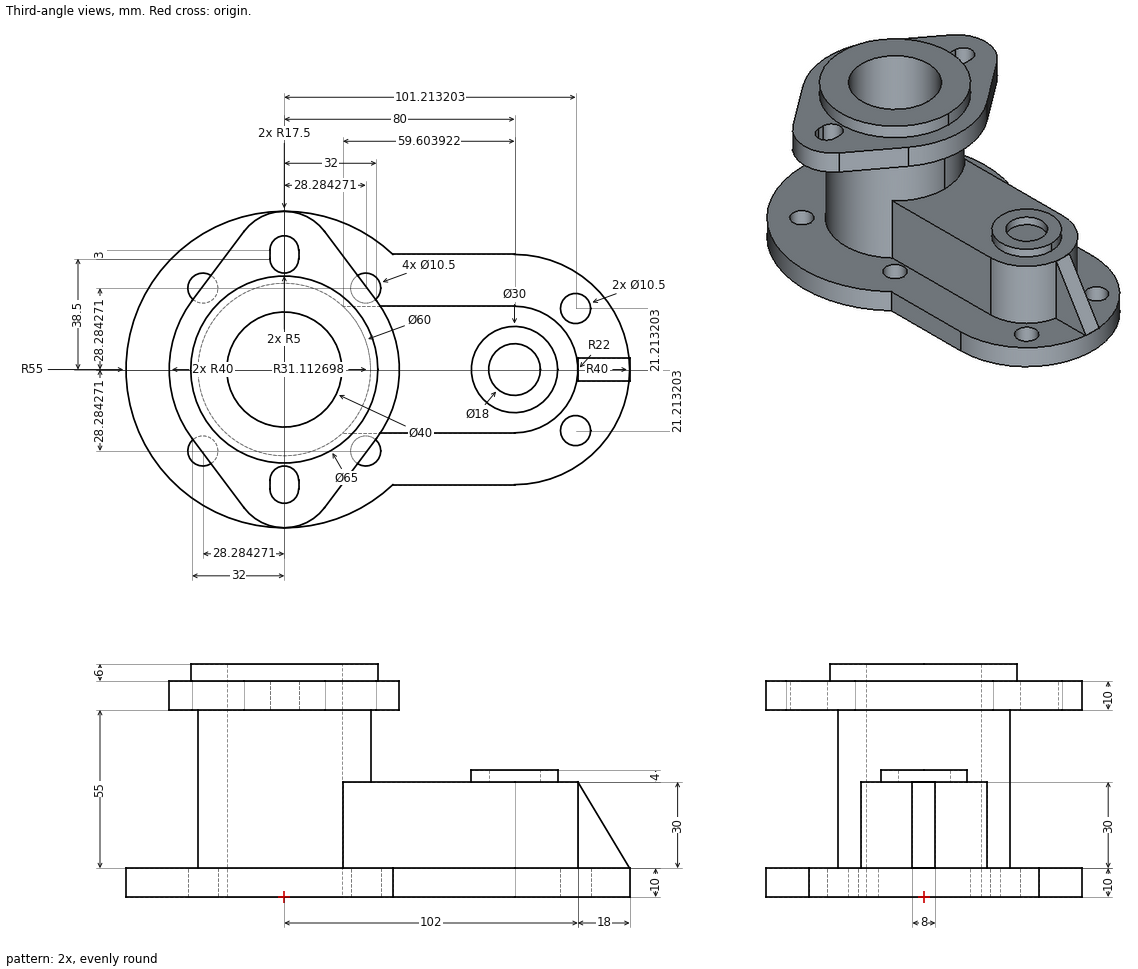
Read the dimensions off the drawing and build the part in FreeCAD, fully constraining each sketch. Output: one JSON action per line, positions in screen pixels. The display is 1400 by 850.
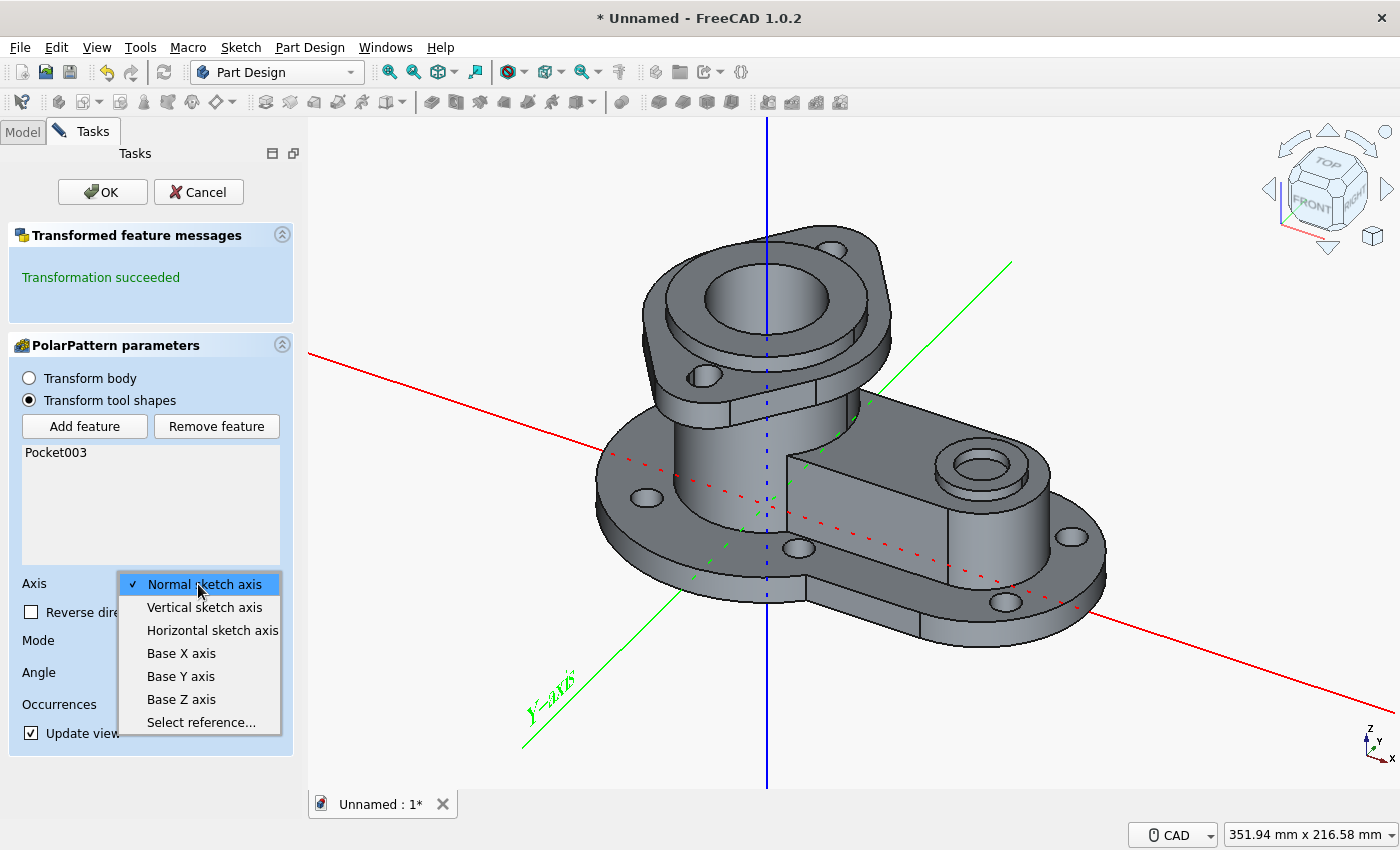
{"action": "left_click", "coordinate": [198, 700]}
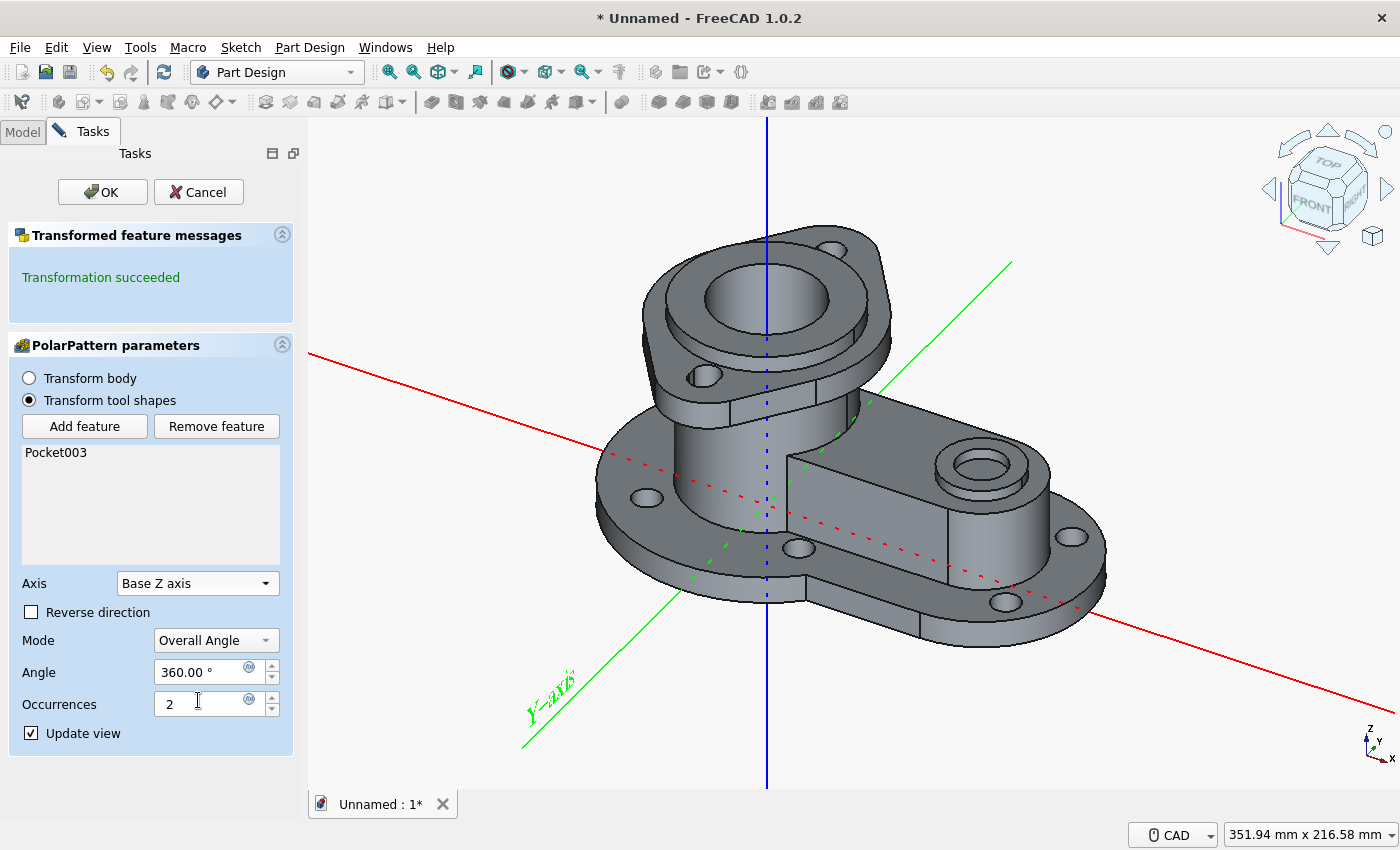
{"action": "triple_click", "coordinate": [209, 704]}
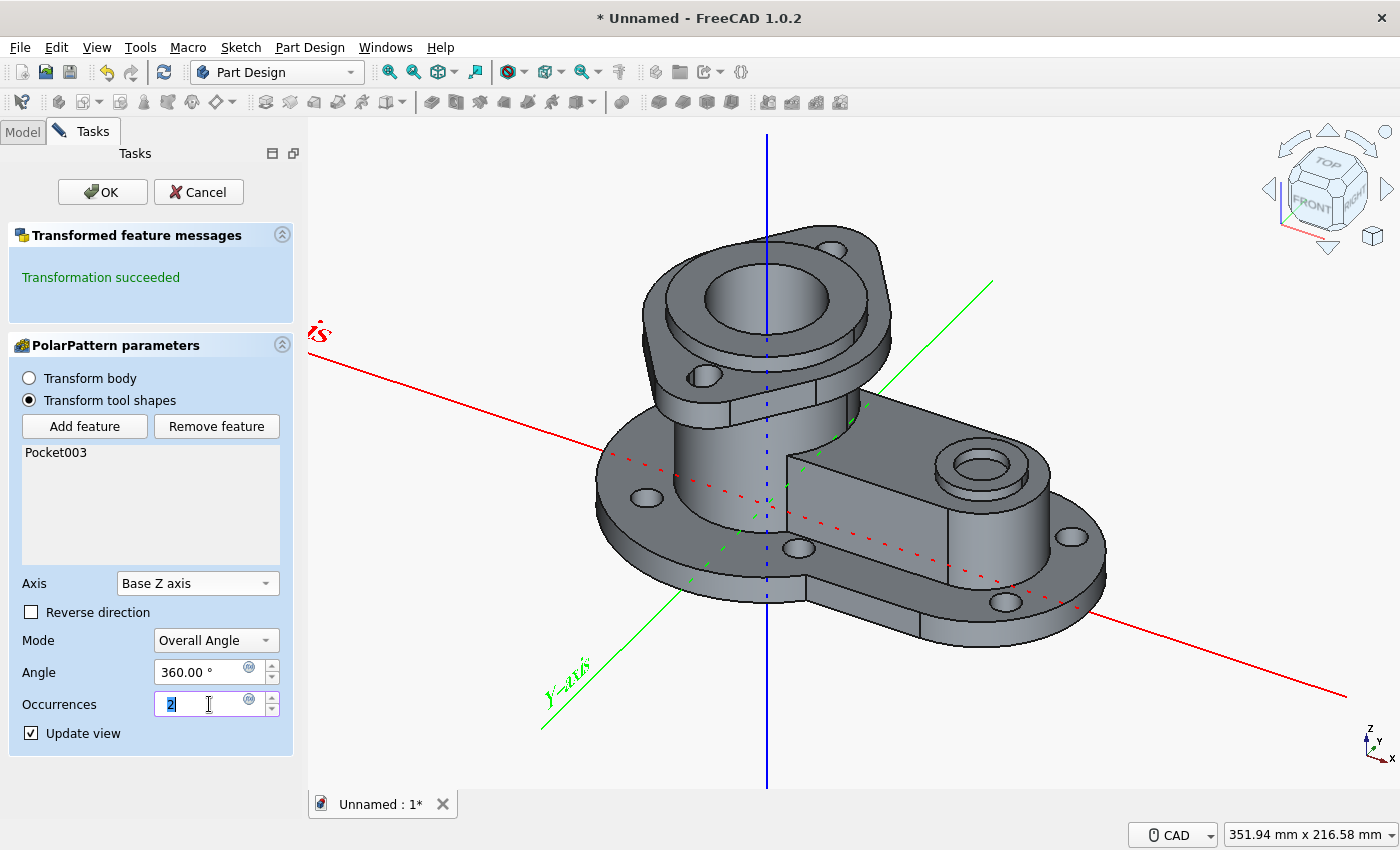
{"action": "type", "text": "2"}
{"action": "key", "text": "Tab"}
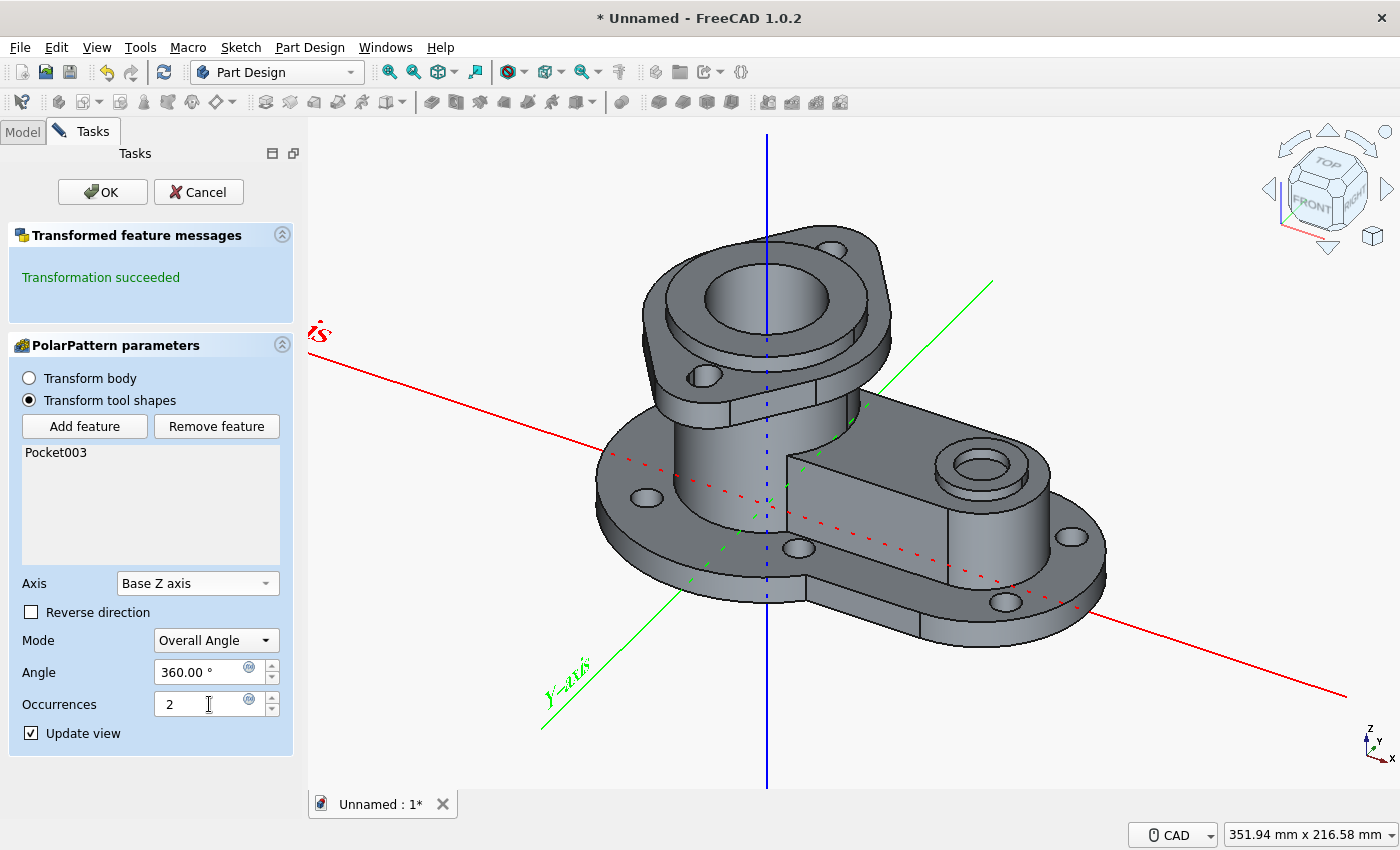
{"action": "left_click", "coordinate": [103, 192]}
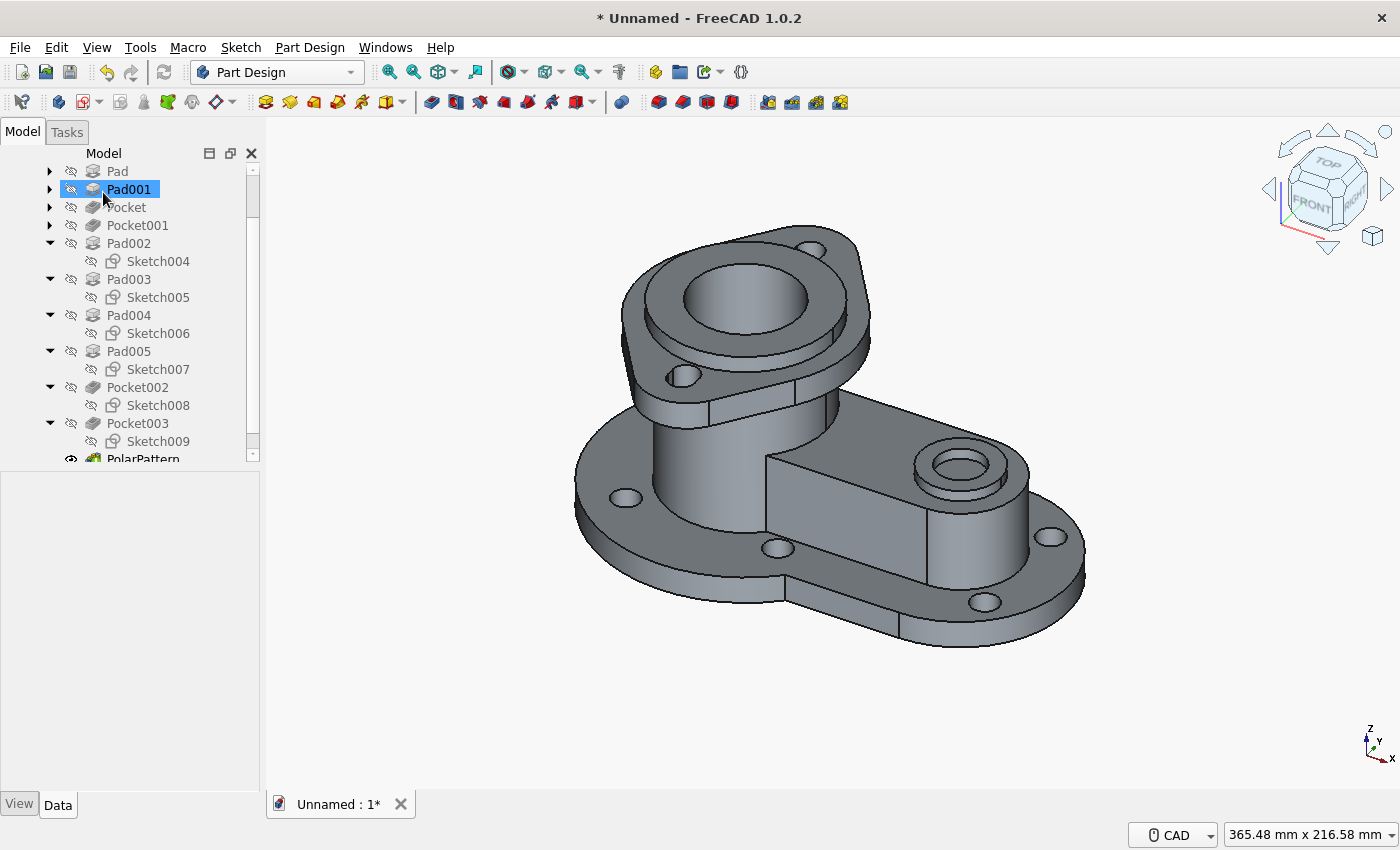
{"action": "left_click", "coordinate": [60, 102]}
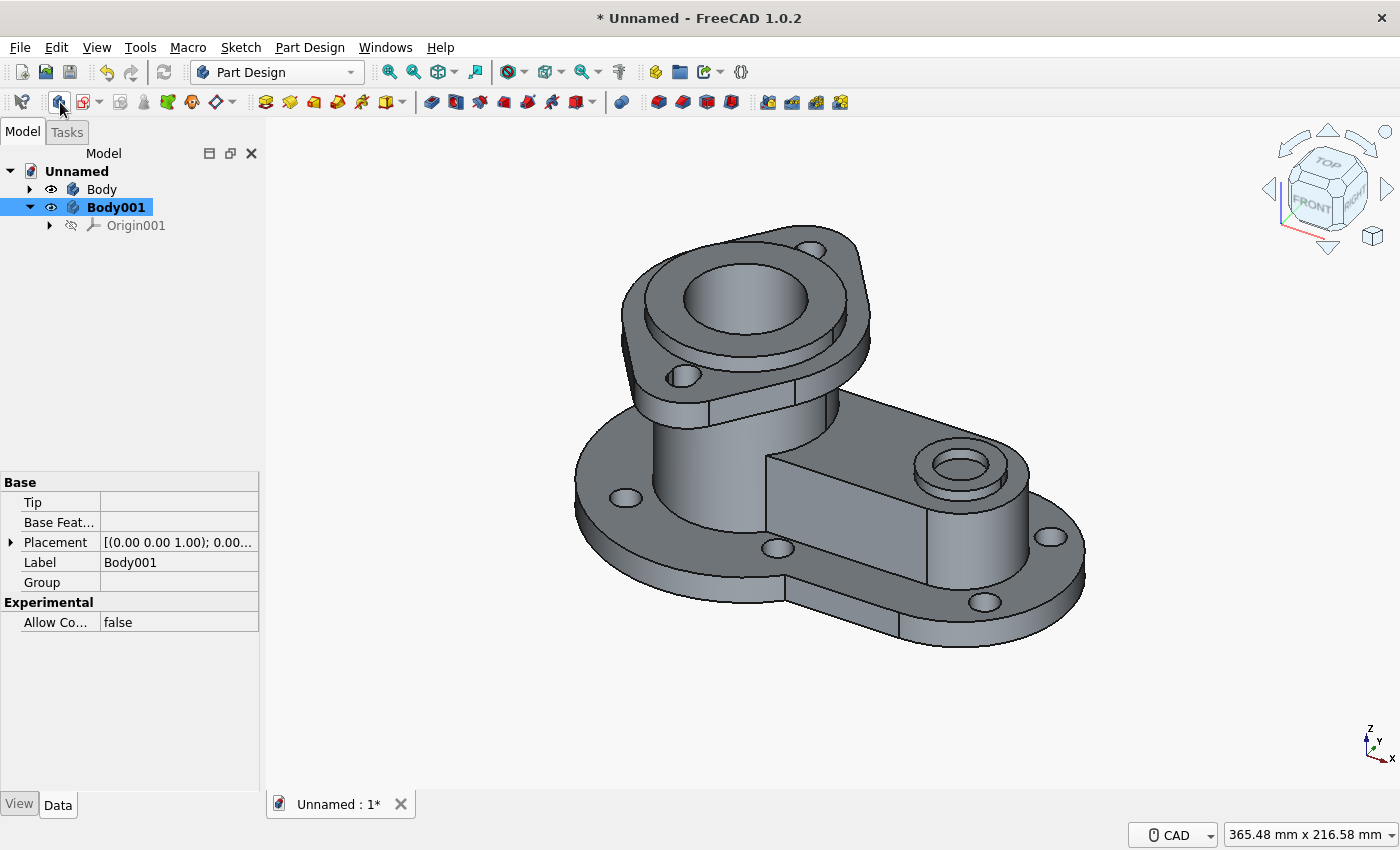
{"action": "left_click", "coordinate": [306, 749]}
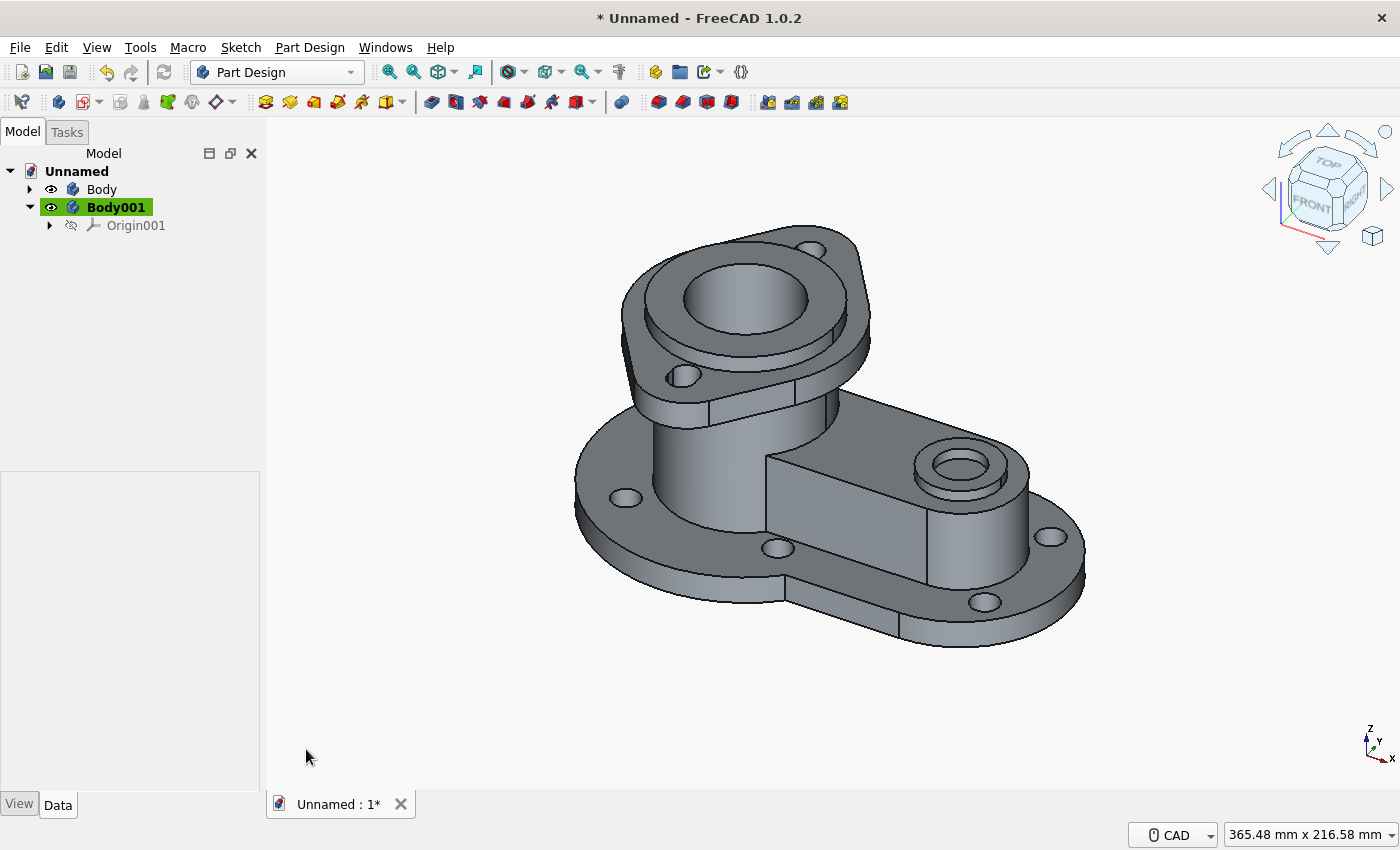
{"action": "left_click", "coordinate": [84, 102]}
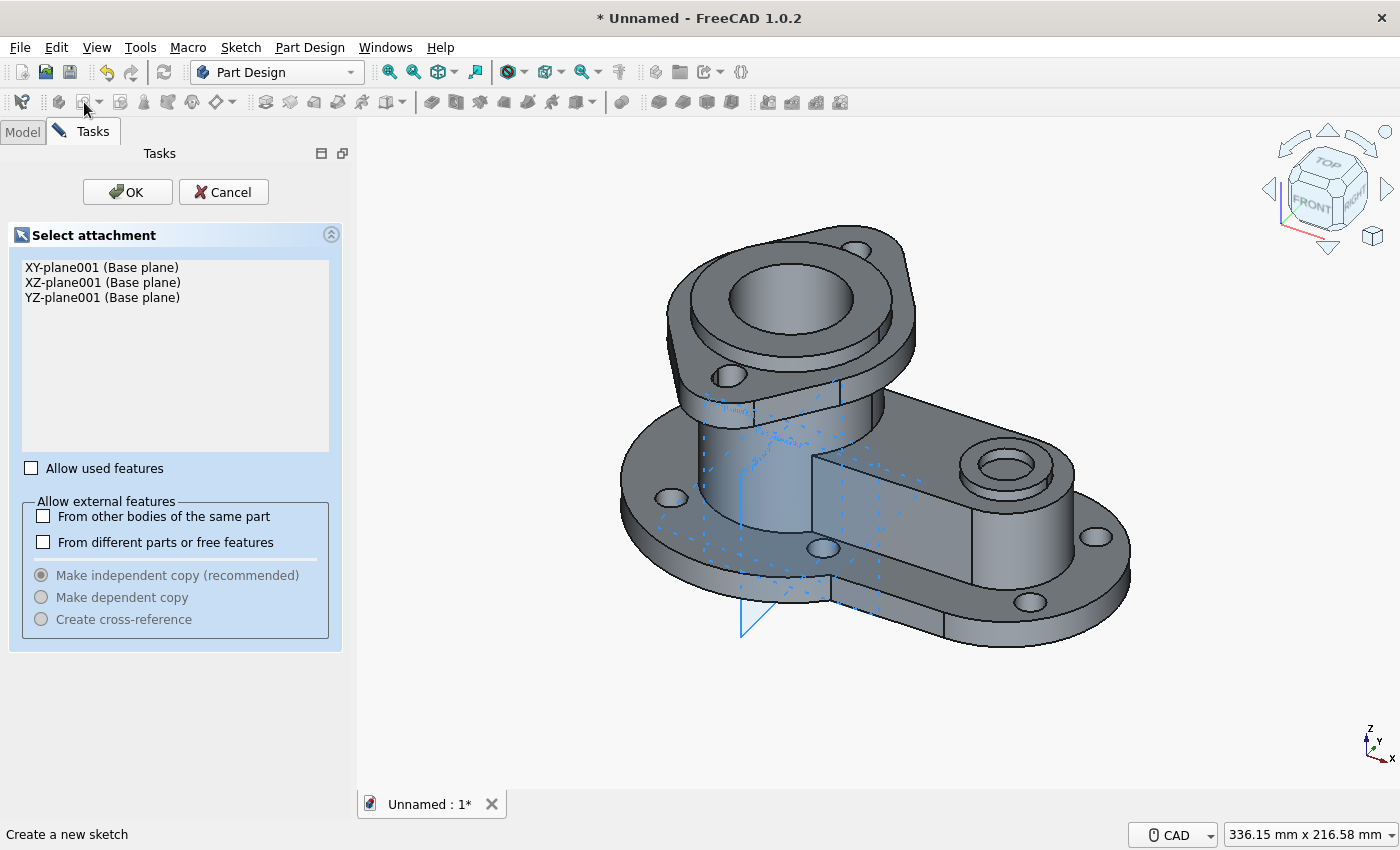
{"action": "left_click", "coordinate": [82, 282]}